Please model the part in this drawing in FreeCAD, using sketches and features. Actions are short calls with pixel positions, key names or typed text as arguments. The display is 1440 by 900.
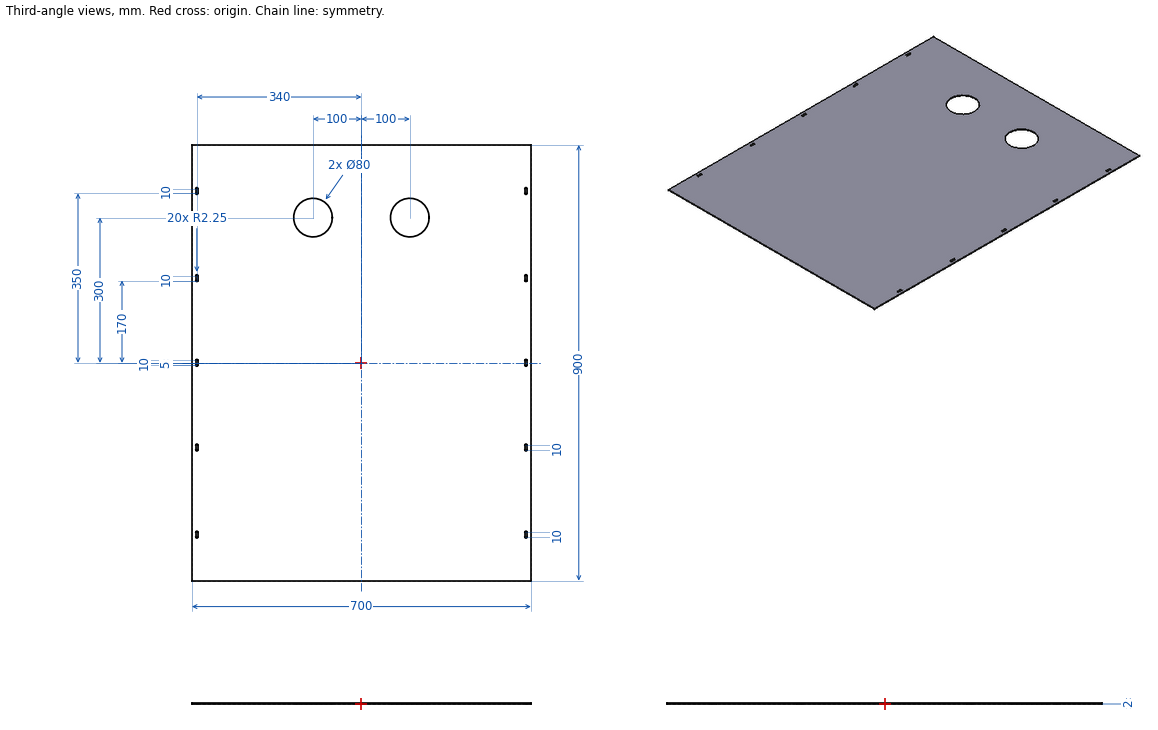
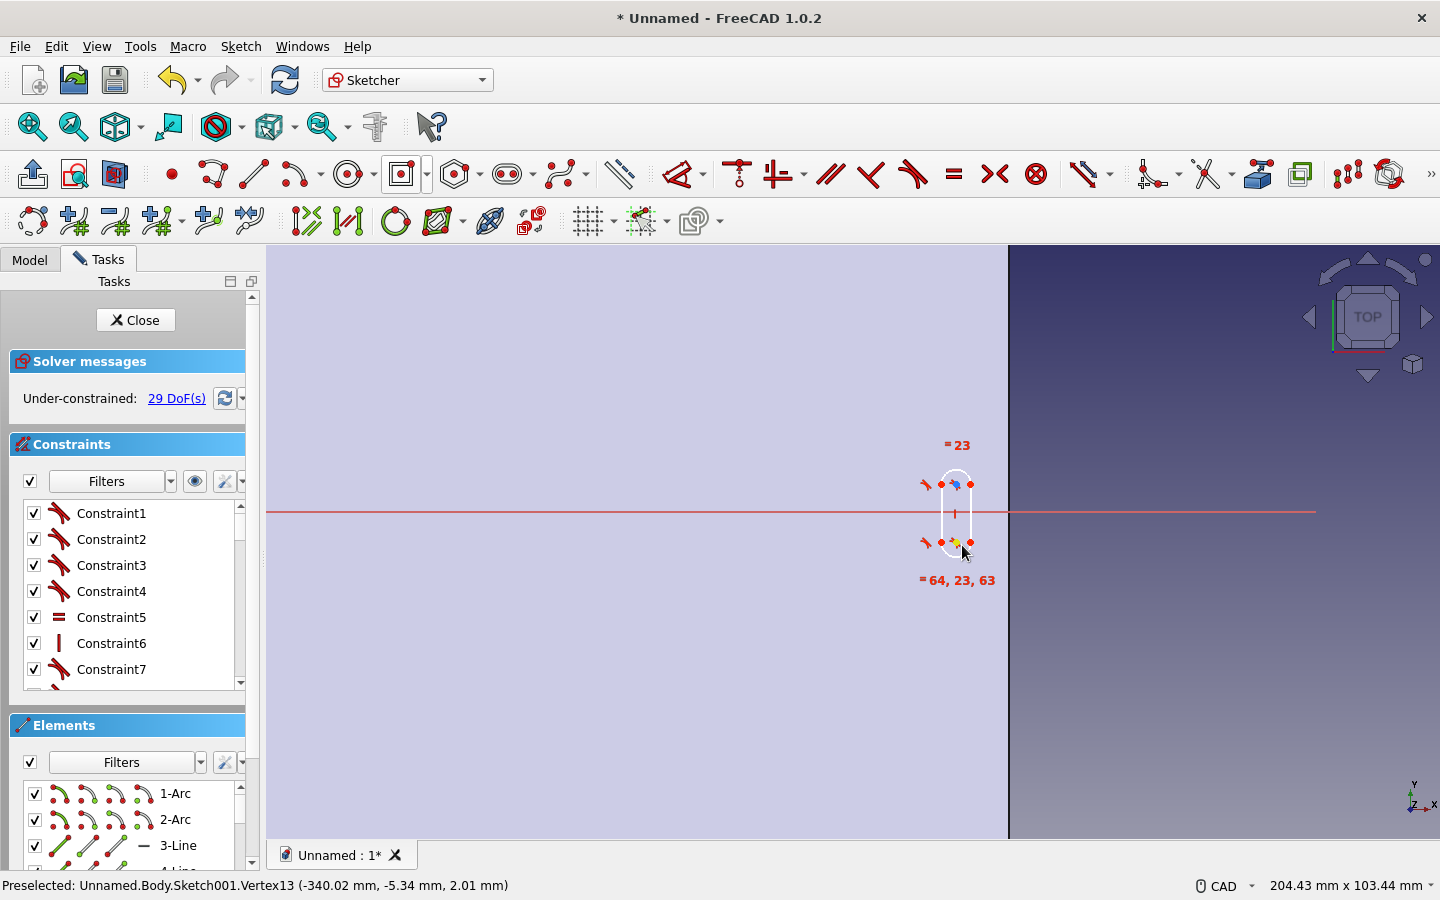
click(956, 543)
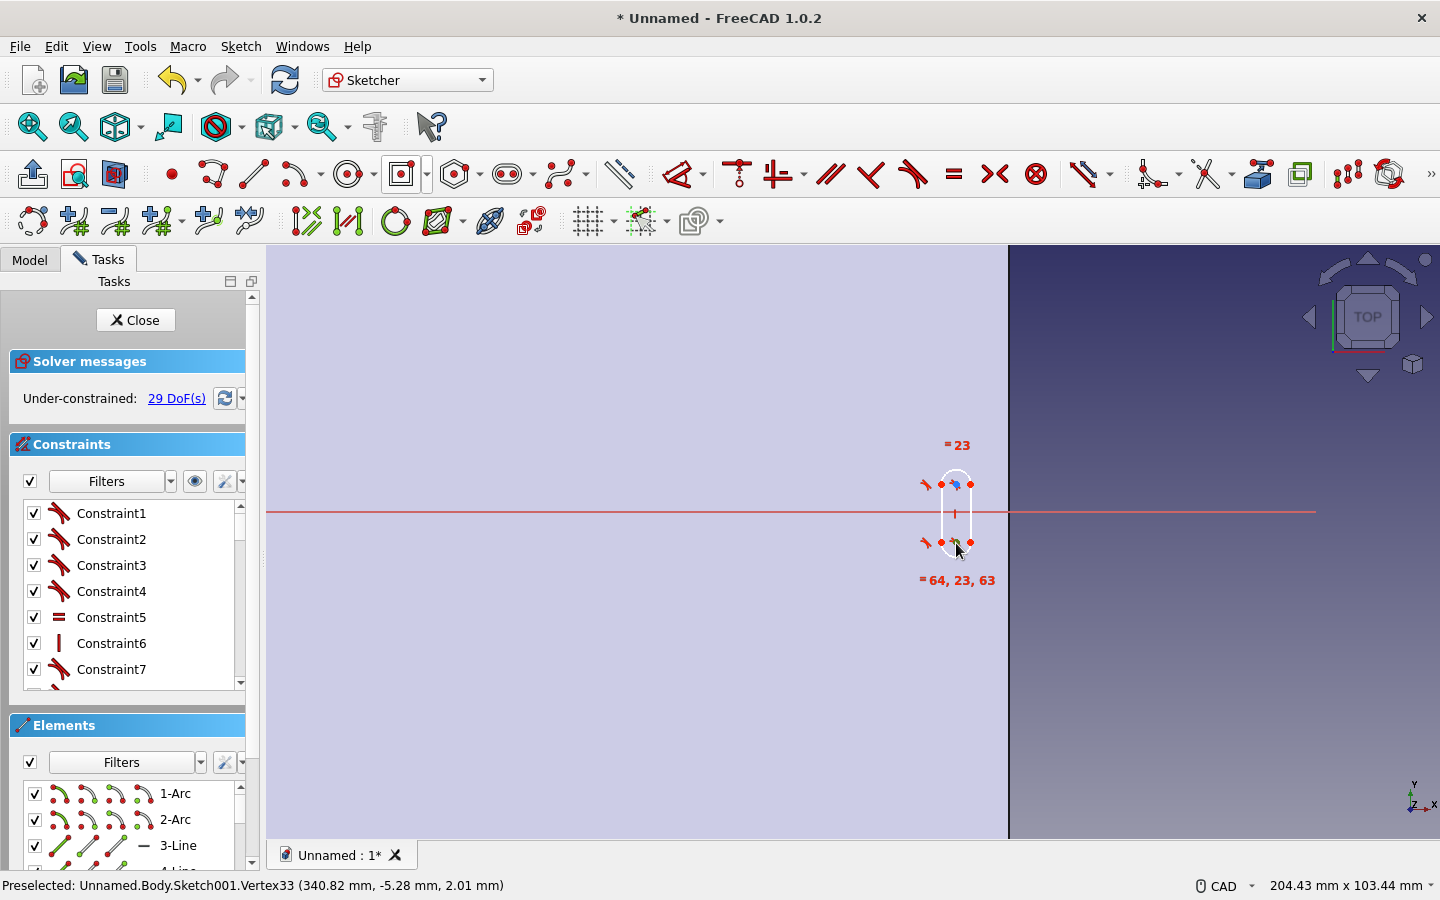
scroll(963, 545, down, 12)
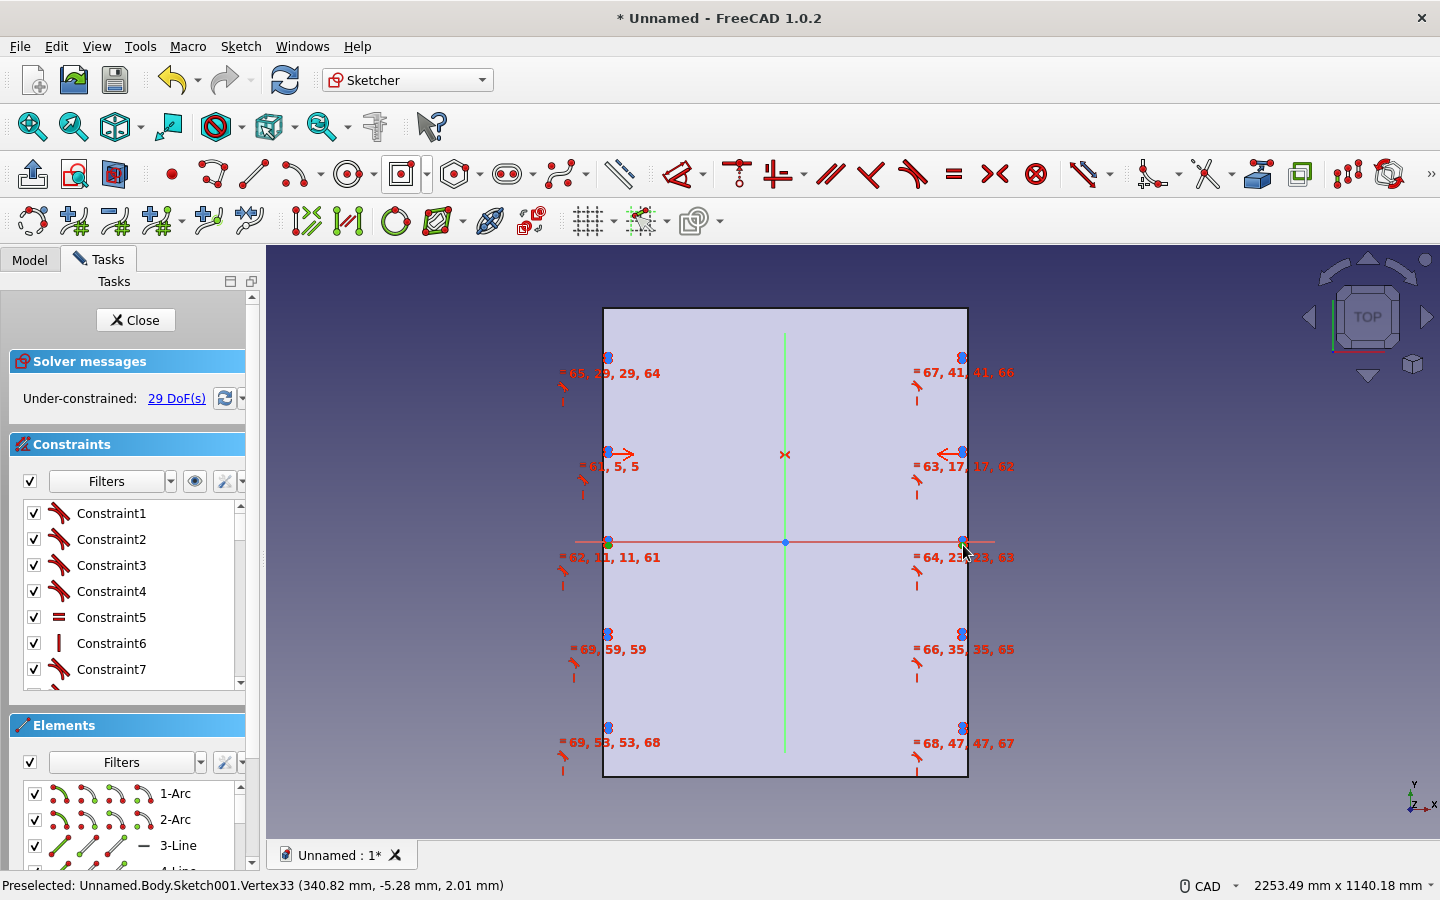
click(785, 734)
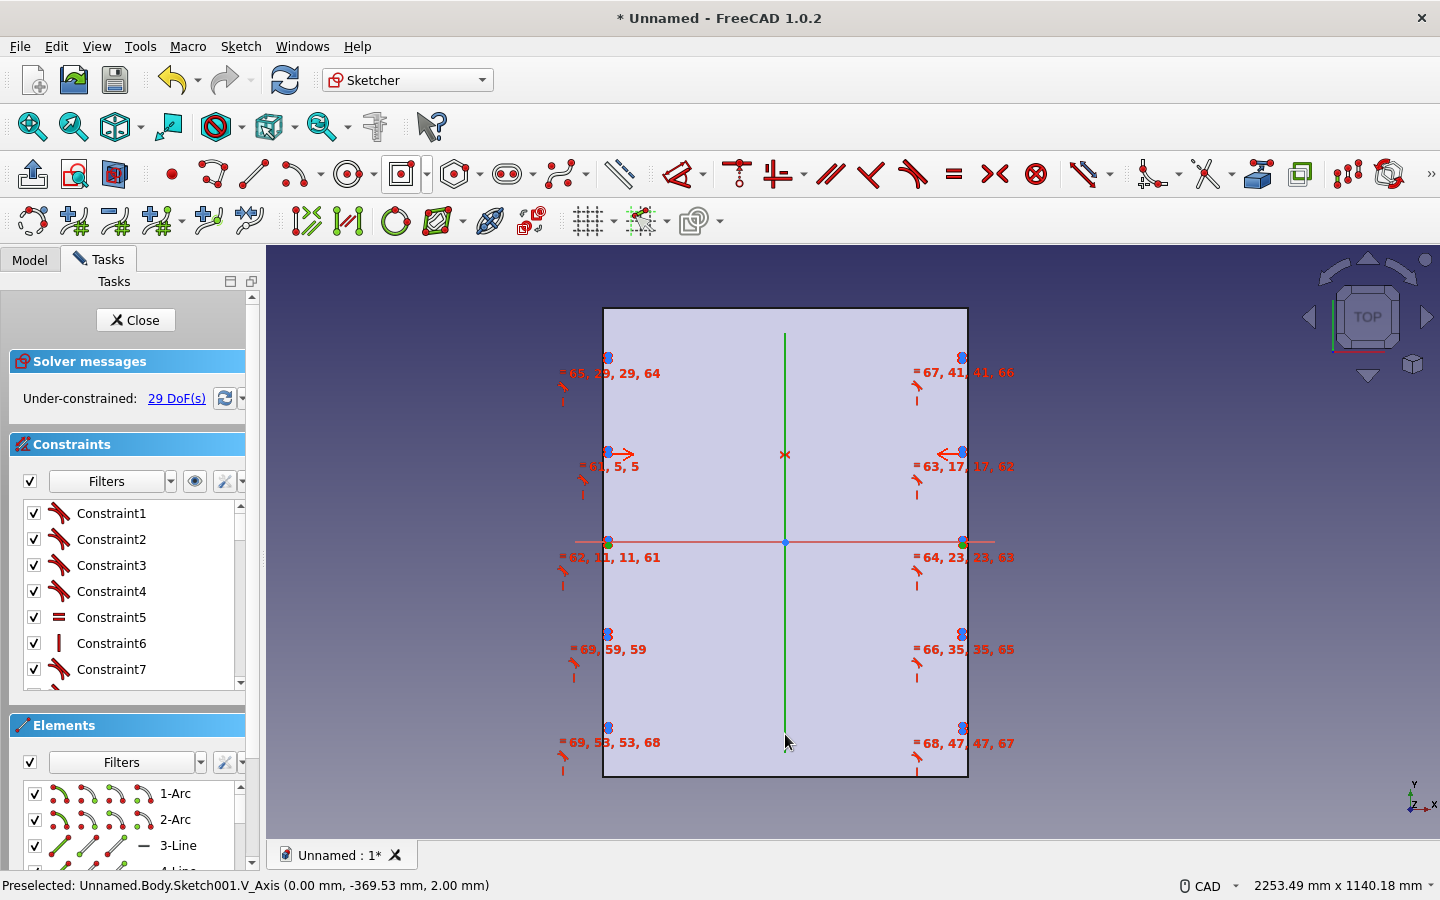
key(s)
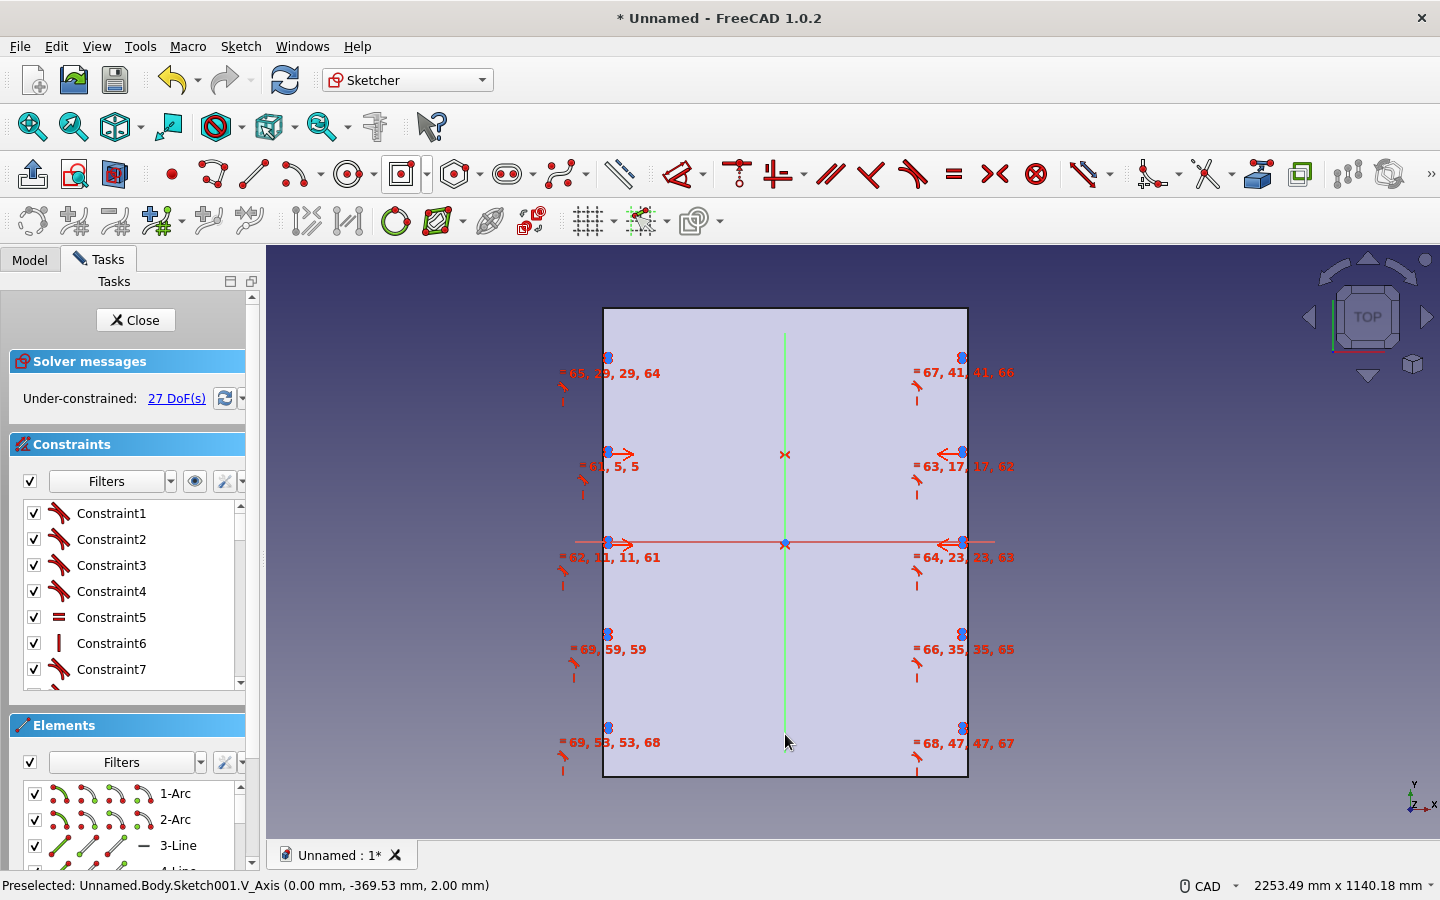
scroll(962, 449, up, 12)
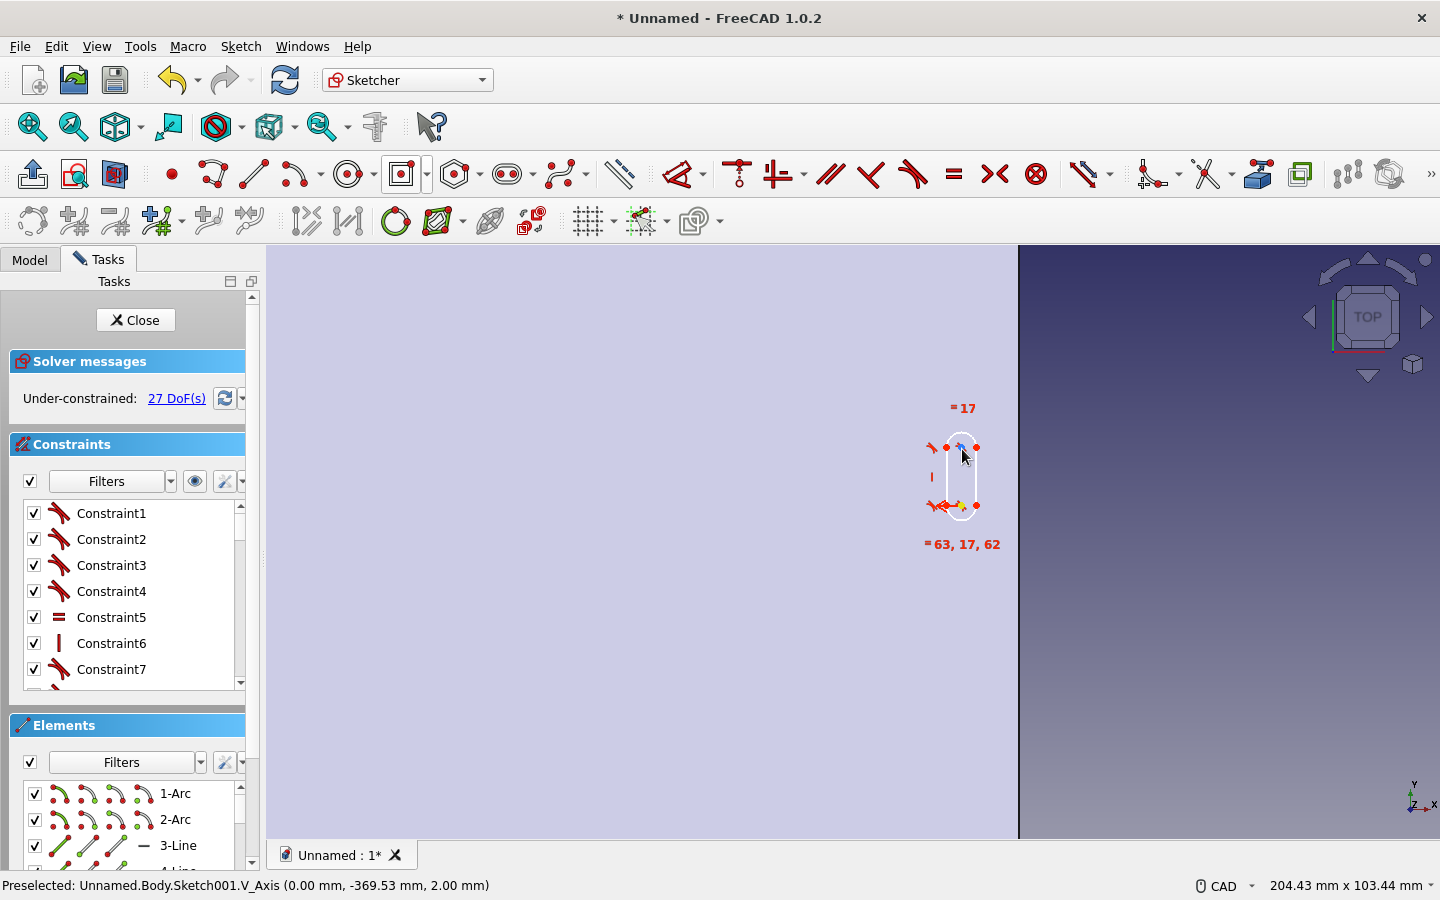
click(962, 447)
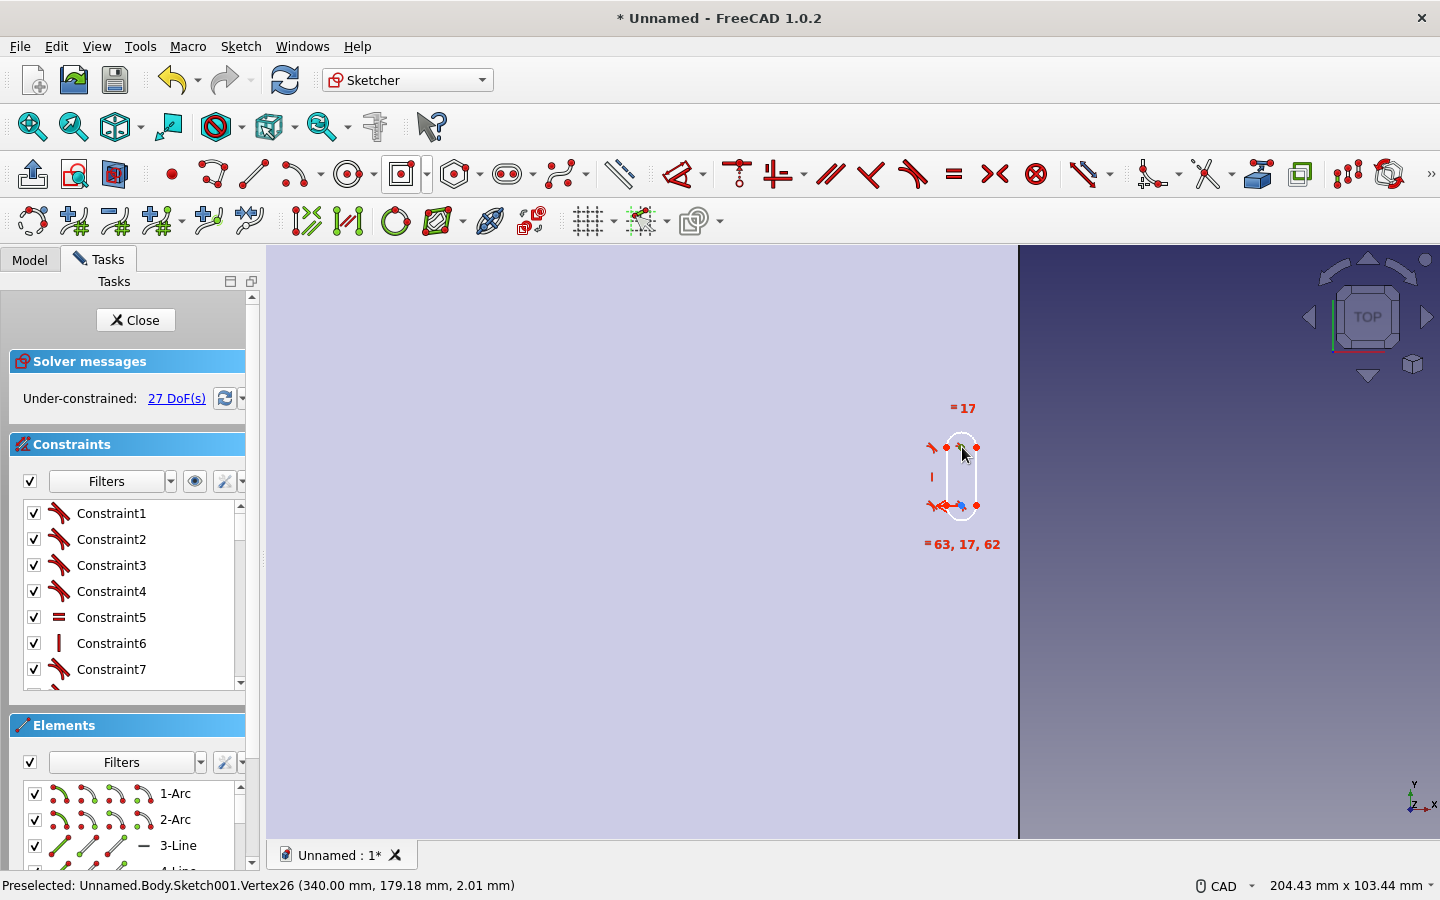
scroll(962, 449, down, 12)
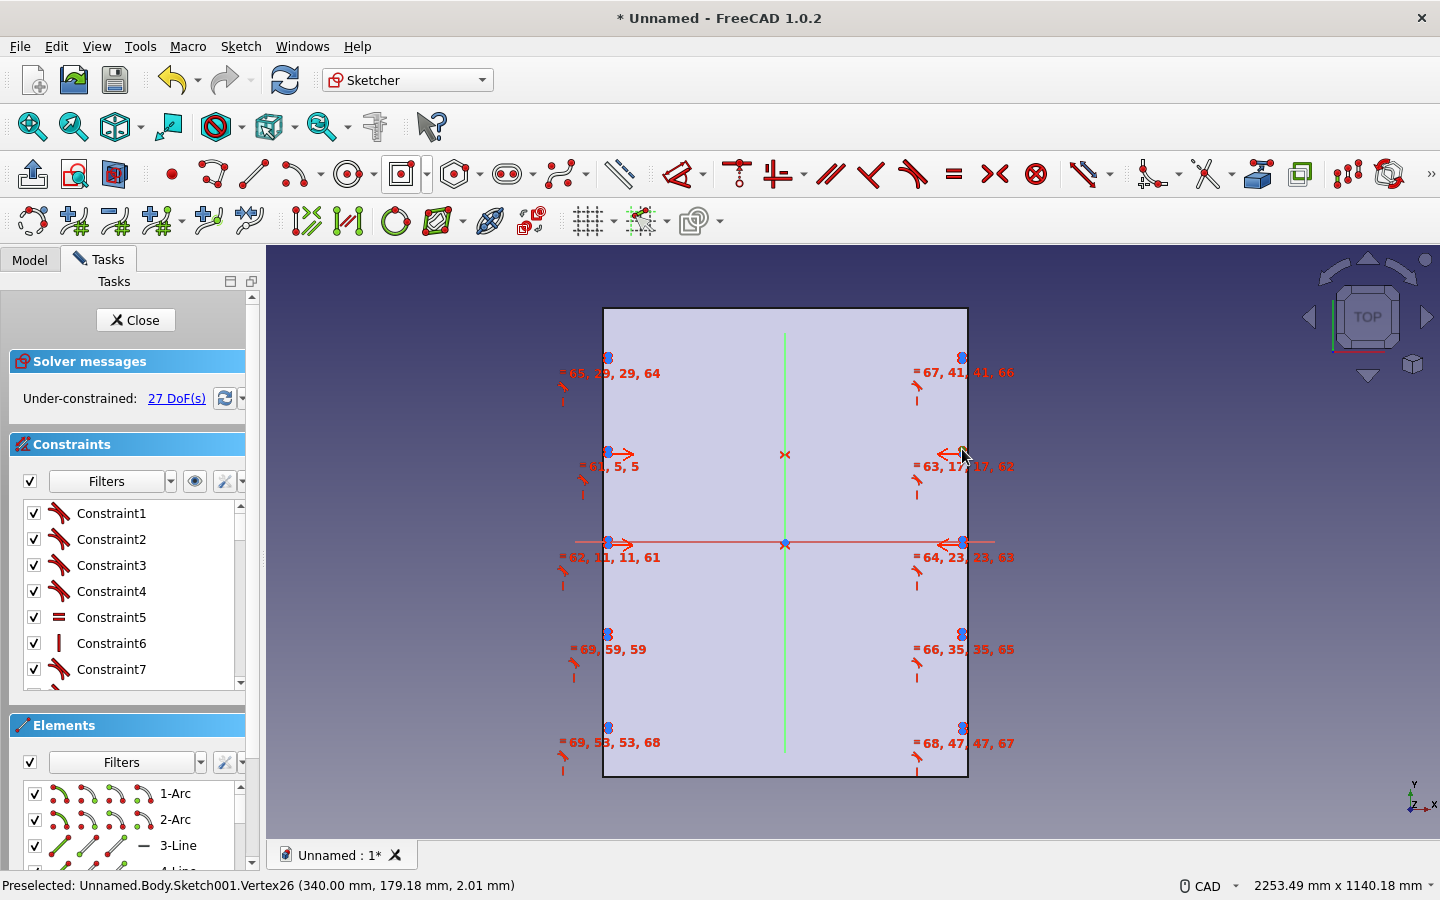
scroll(962, 637, up, 12)